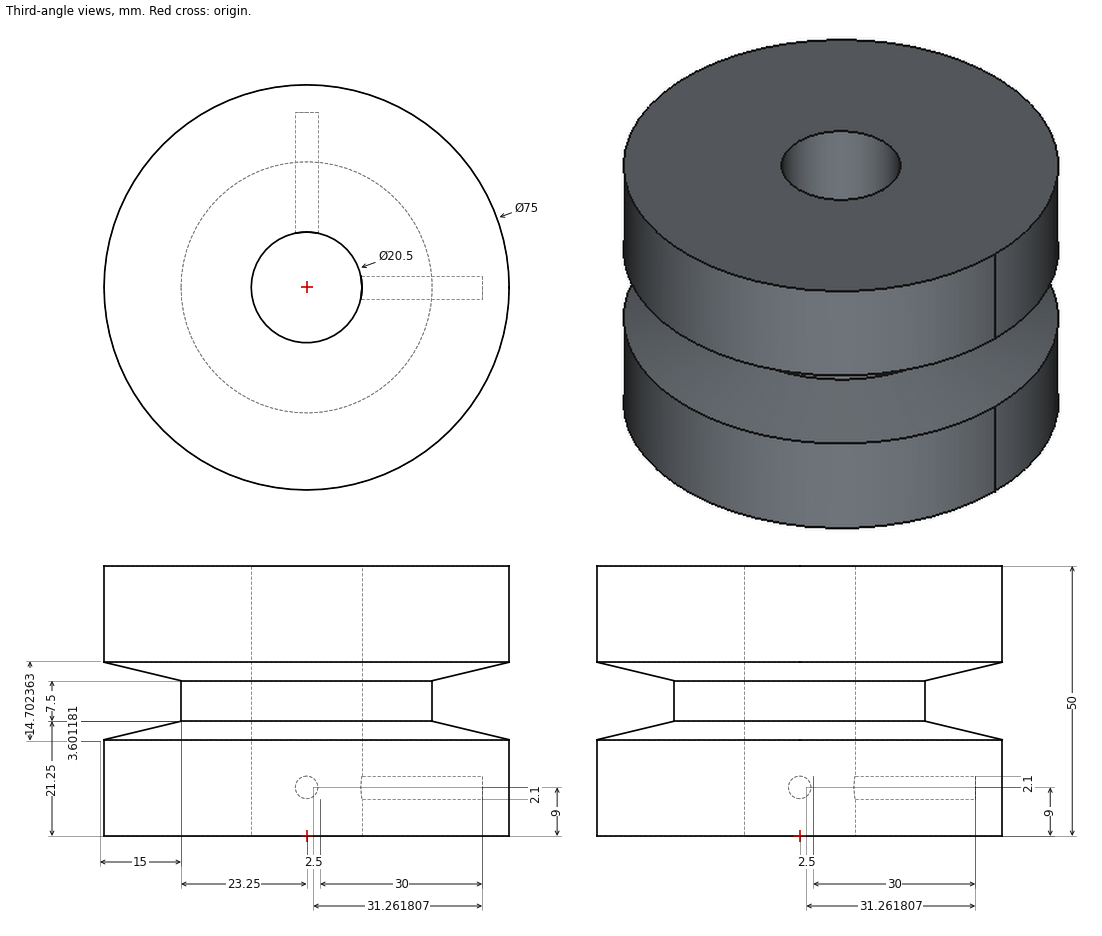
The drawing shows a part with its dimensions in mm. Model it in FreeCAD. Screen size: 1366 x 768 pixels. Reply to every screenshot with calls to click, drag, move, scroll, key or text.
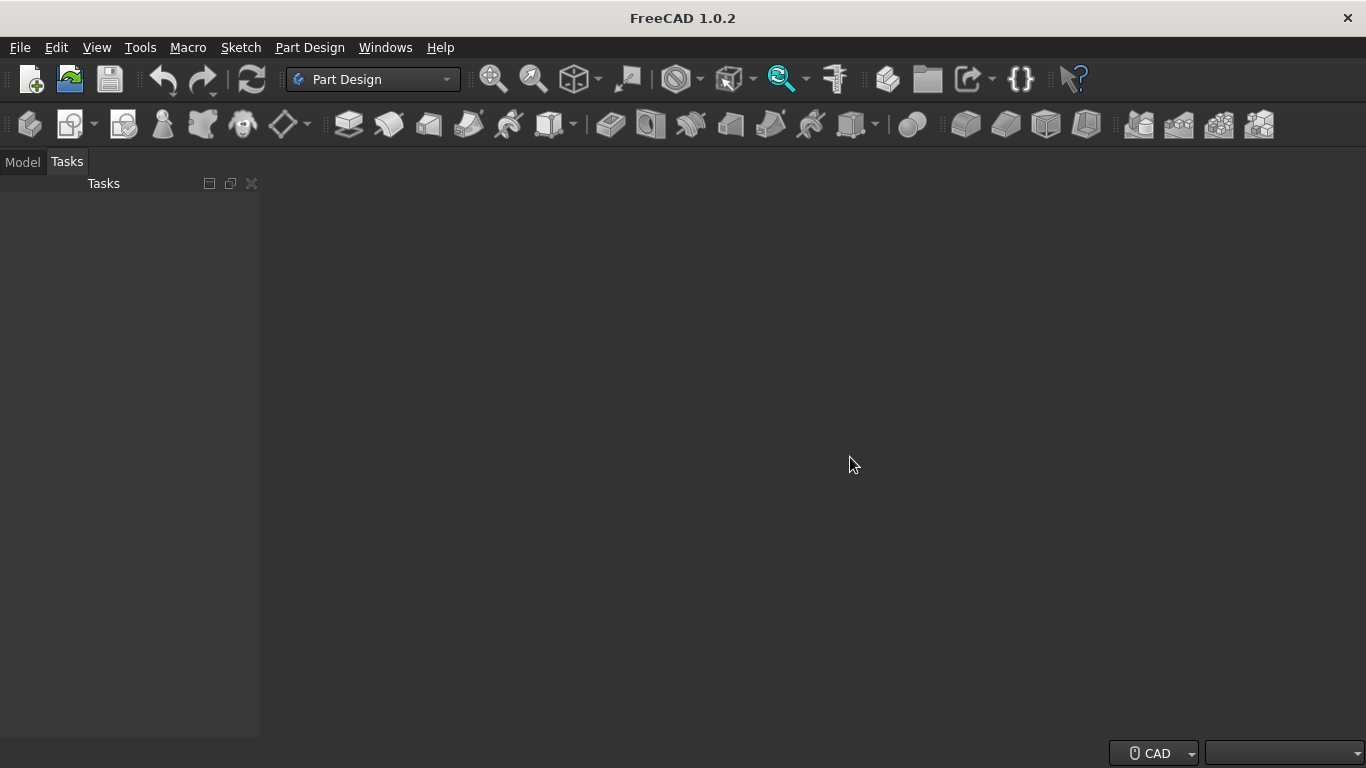
key(ctrl+n)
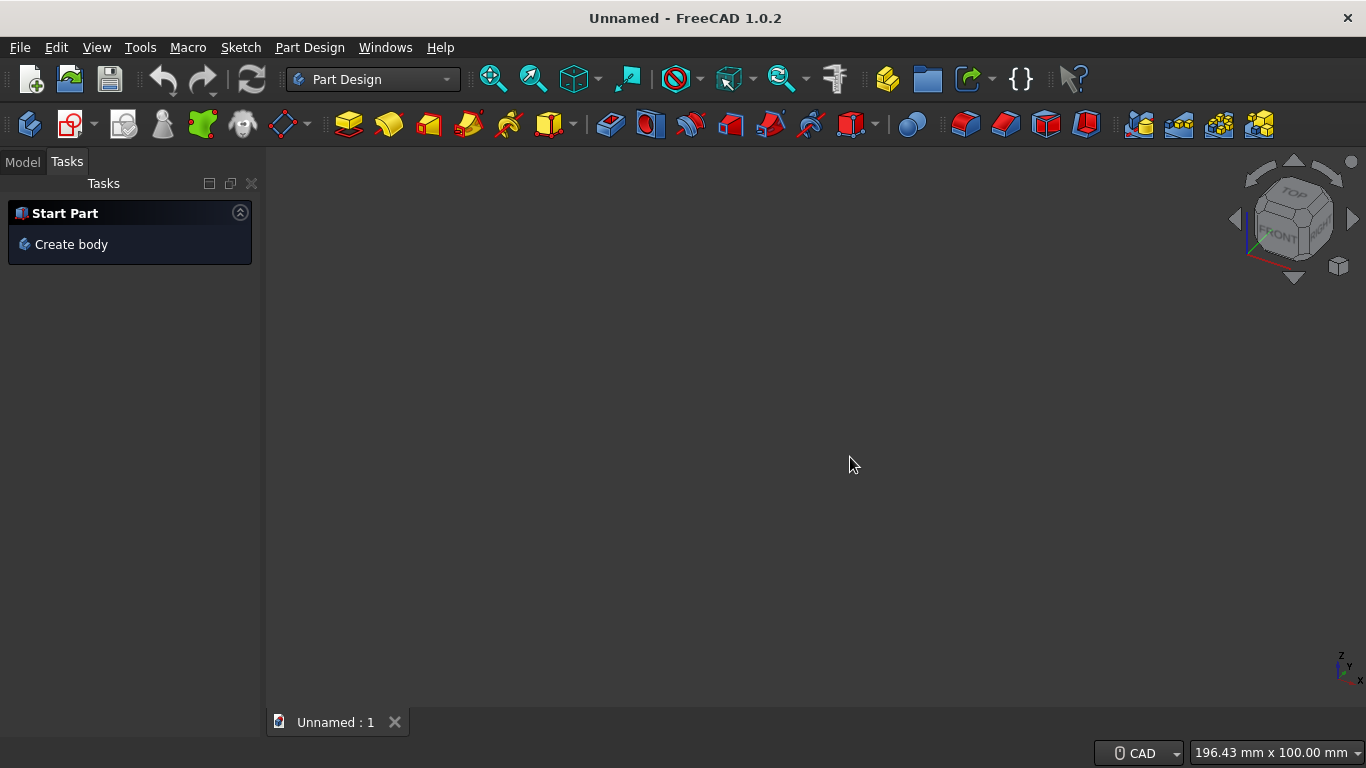
click(70, 124)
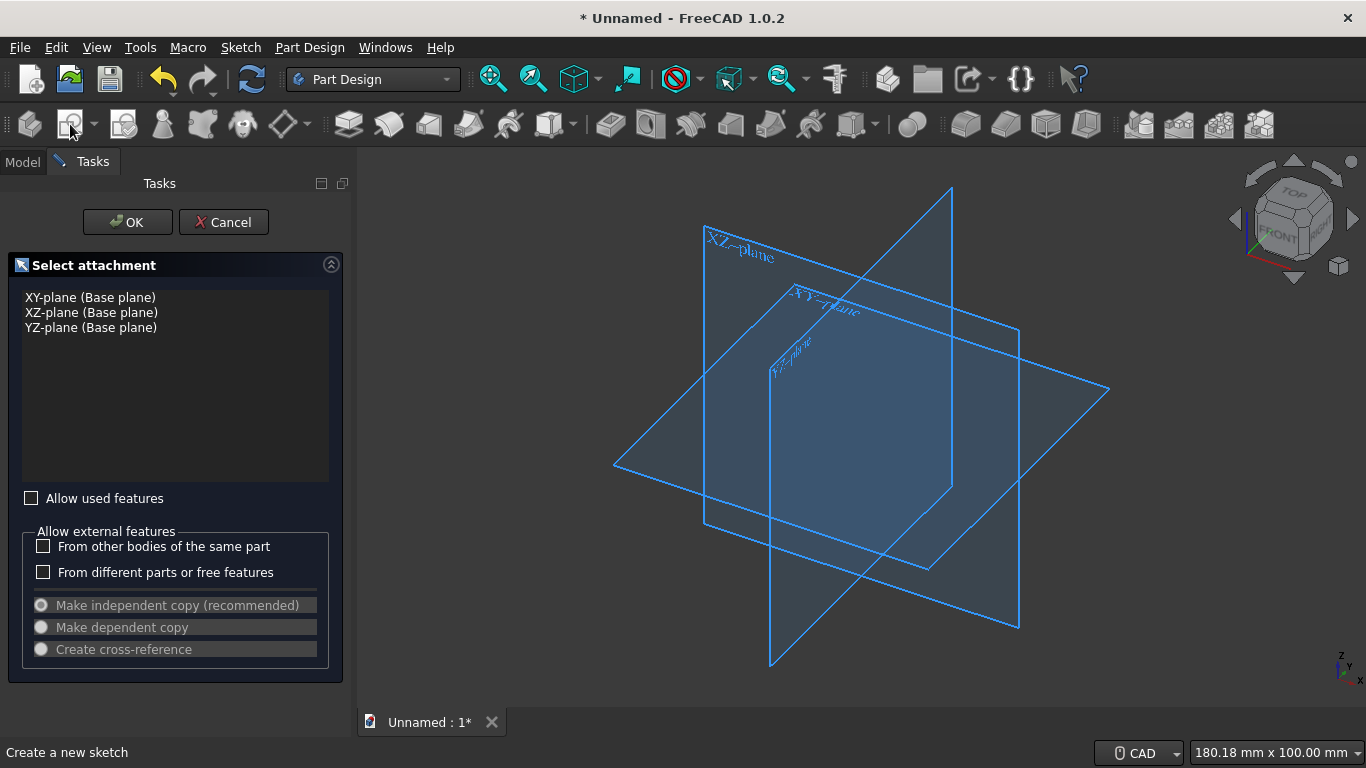
click(82, 298)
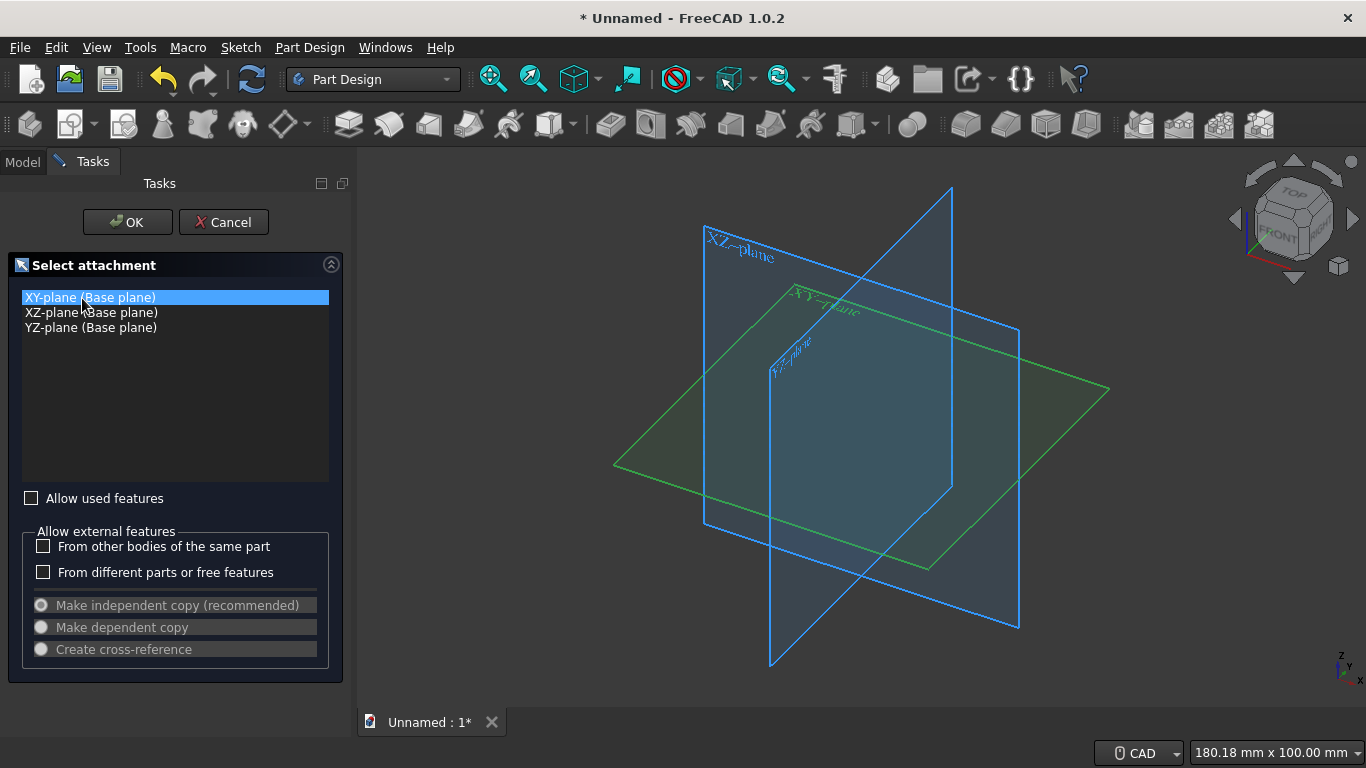
click(128, 222)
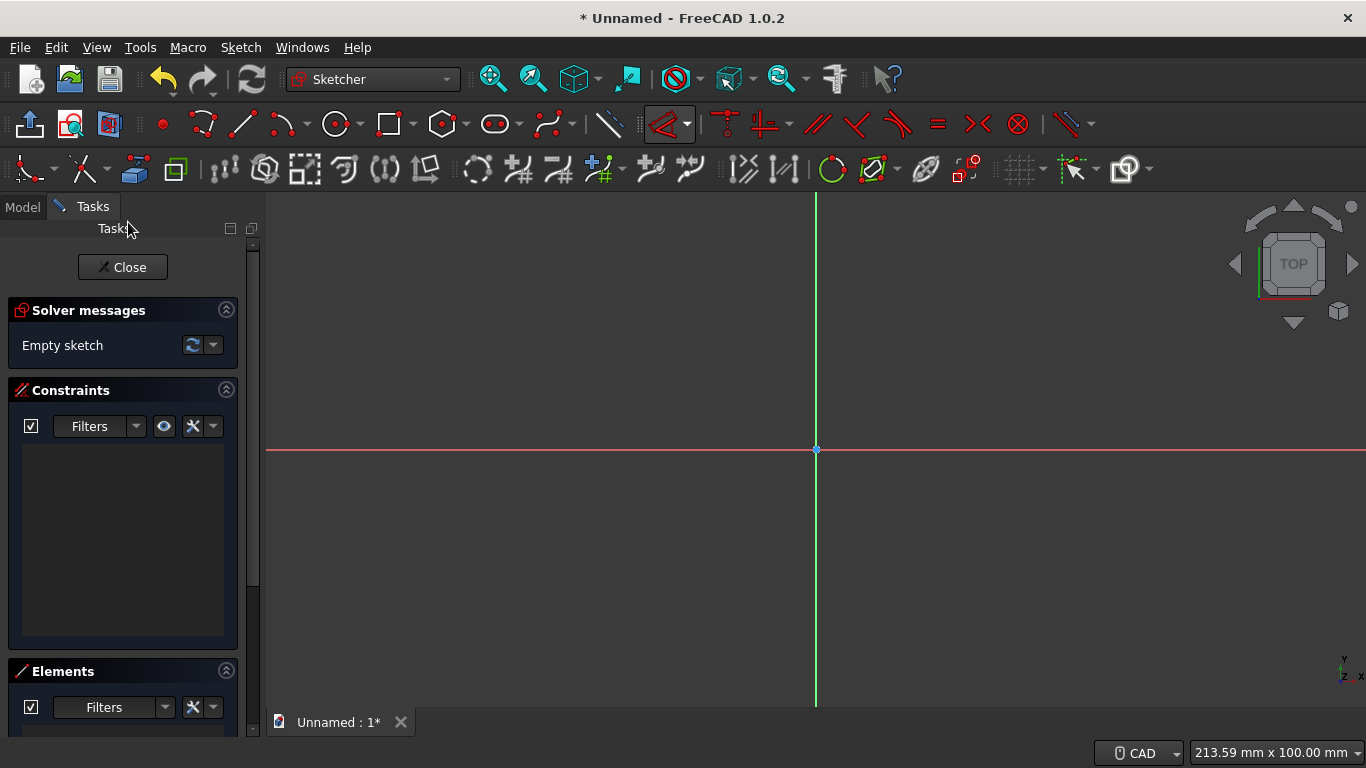
key(g)
key(c)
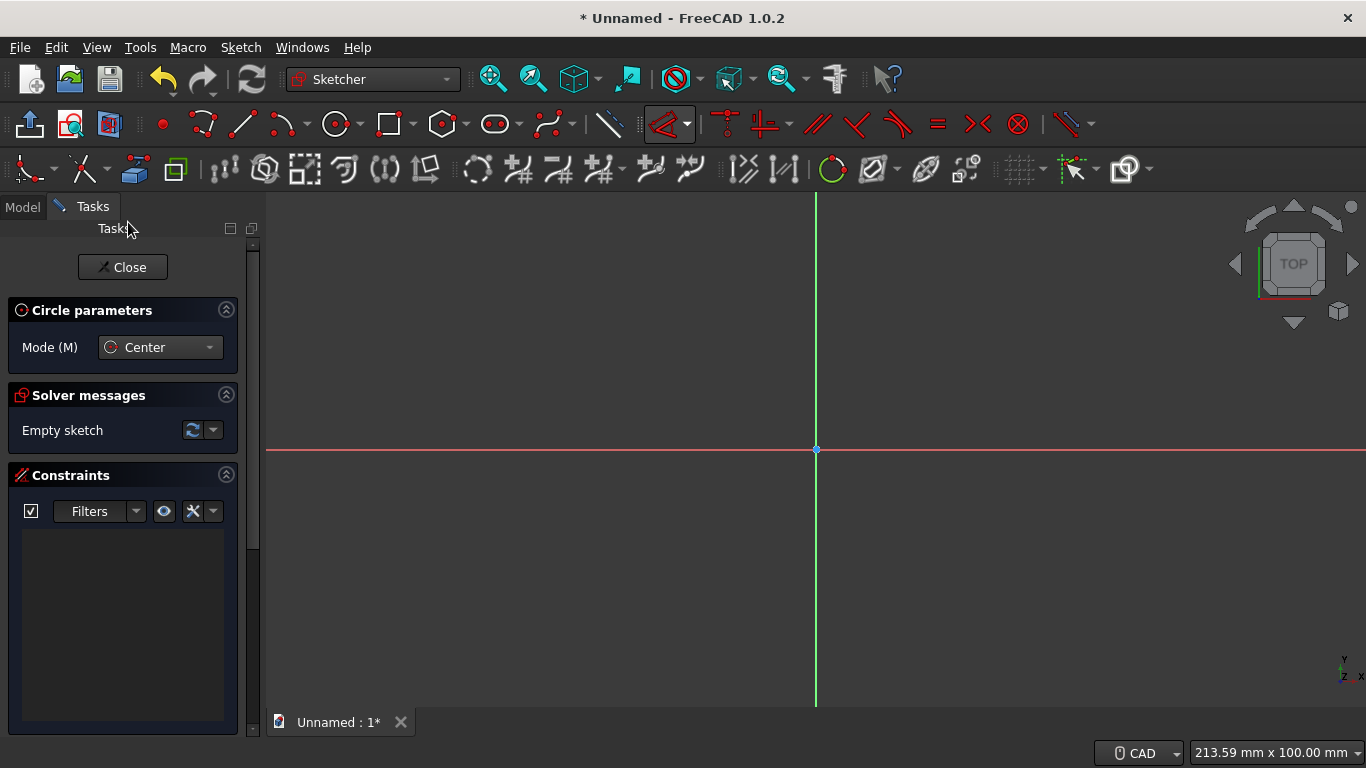
click(816, 450)
move(953, 313)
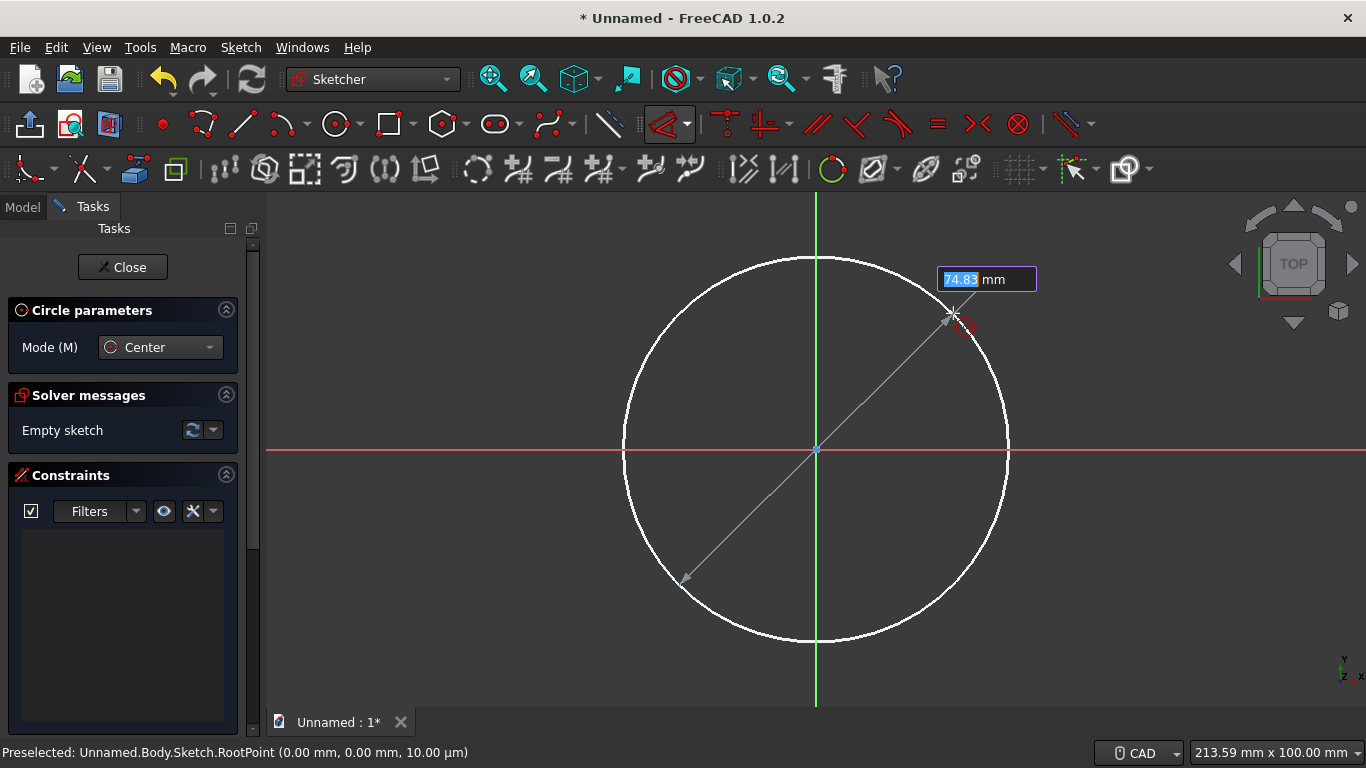
text(75)
key(Return)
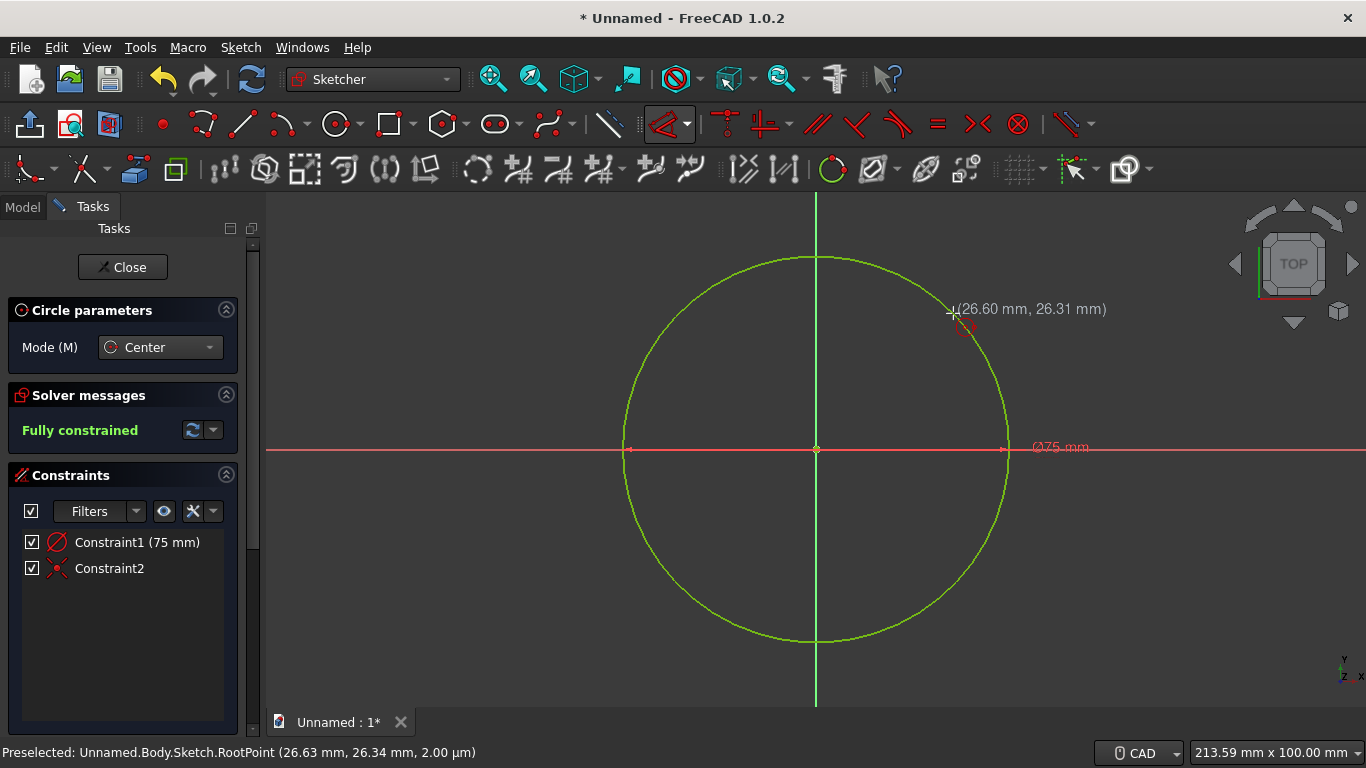
click(816, 450)
move(853, 412)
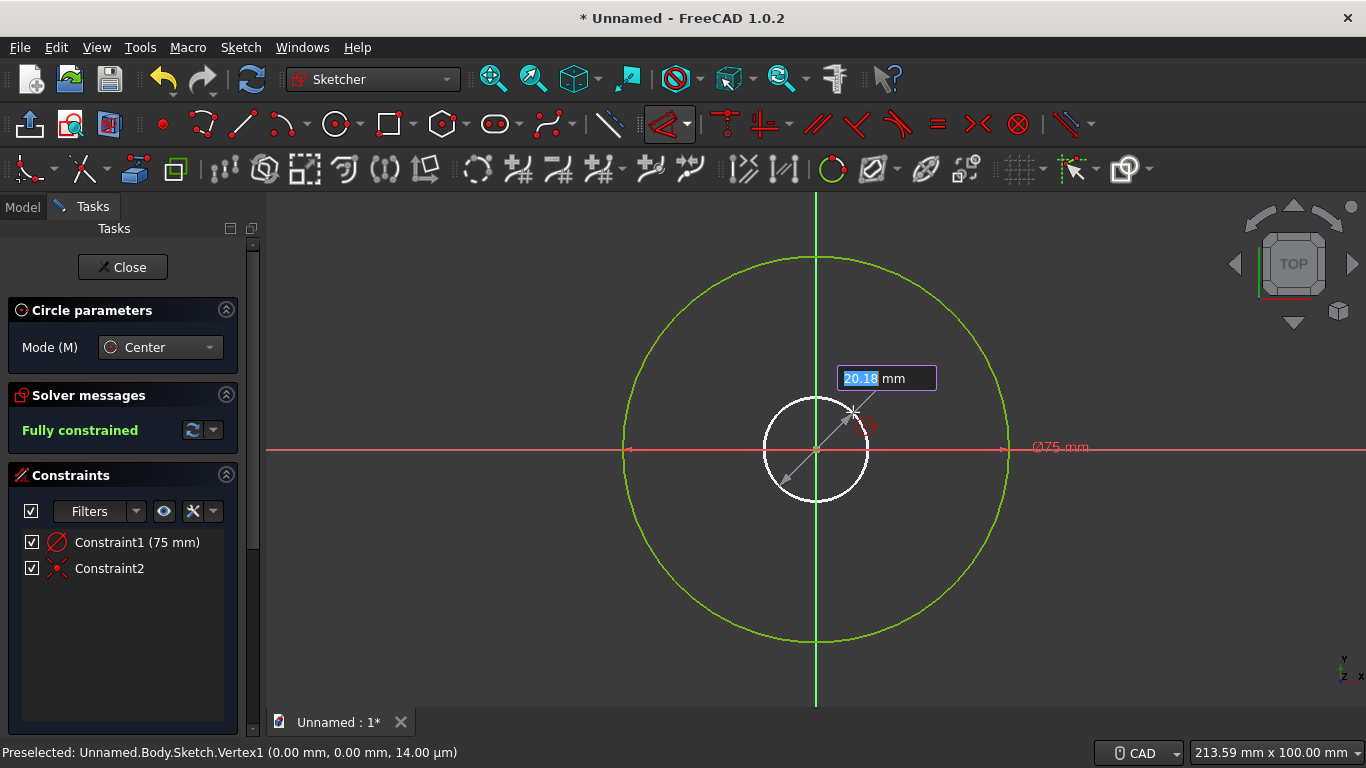
text(20.5)
key(Return)
key(Escape)